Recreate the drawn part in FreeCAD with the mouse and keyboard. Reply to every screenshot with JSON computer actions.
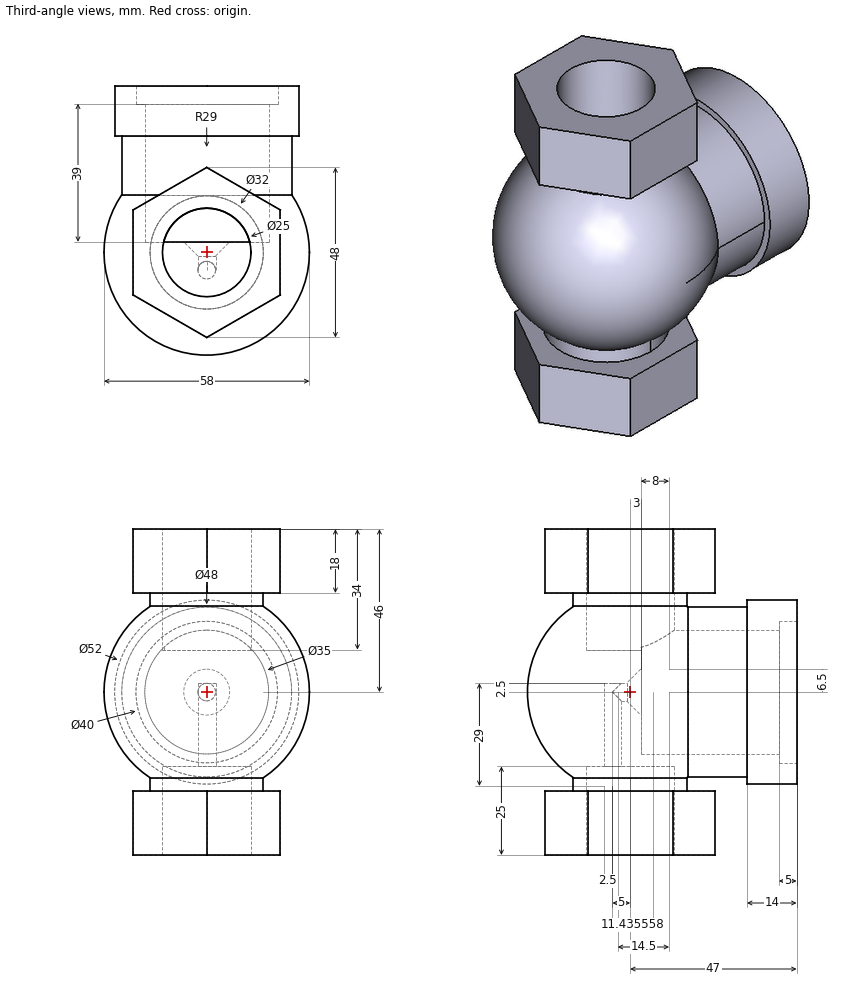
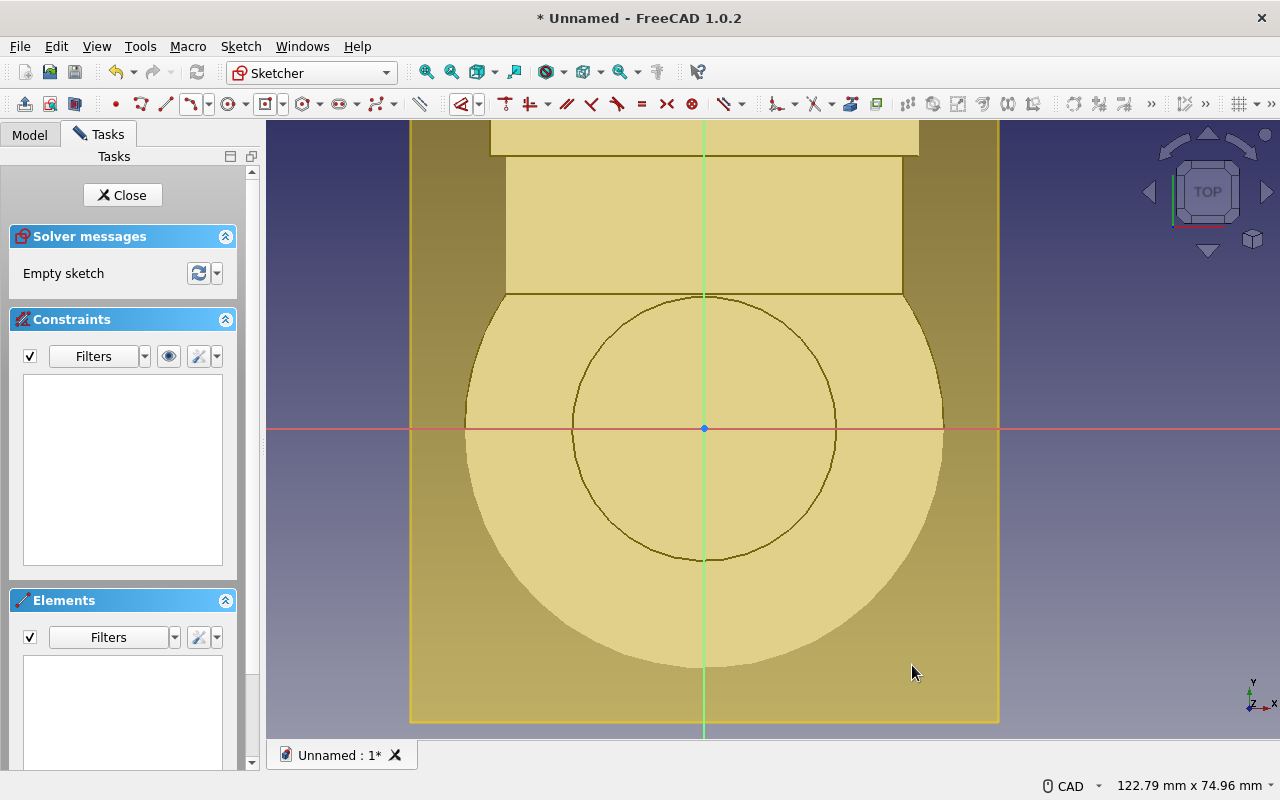
{"action": "left_click", "coordinate": [302, 104]}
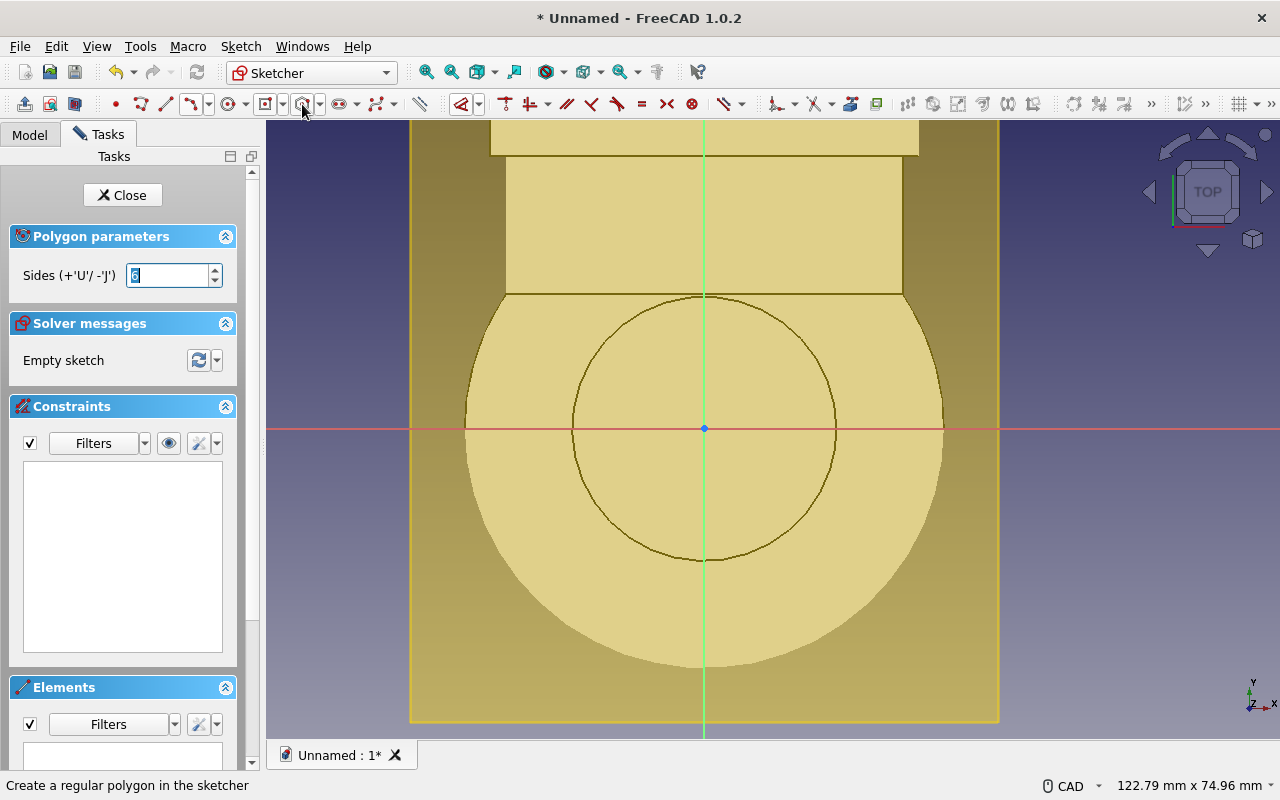
{"action": "left_click", "coordinate": [704, 429]}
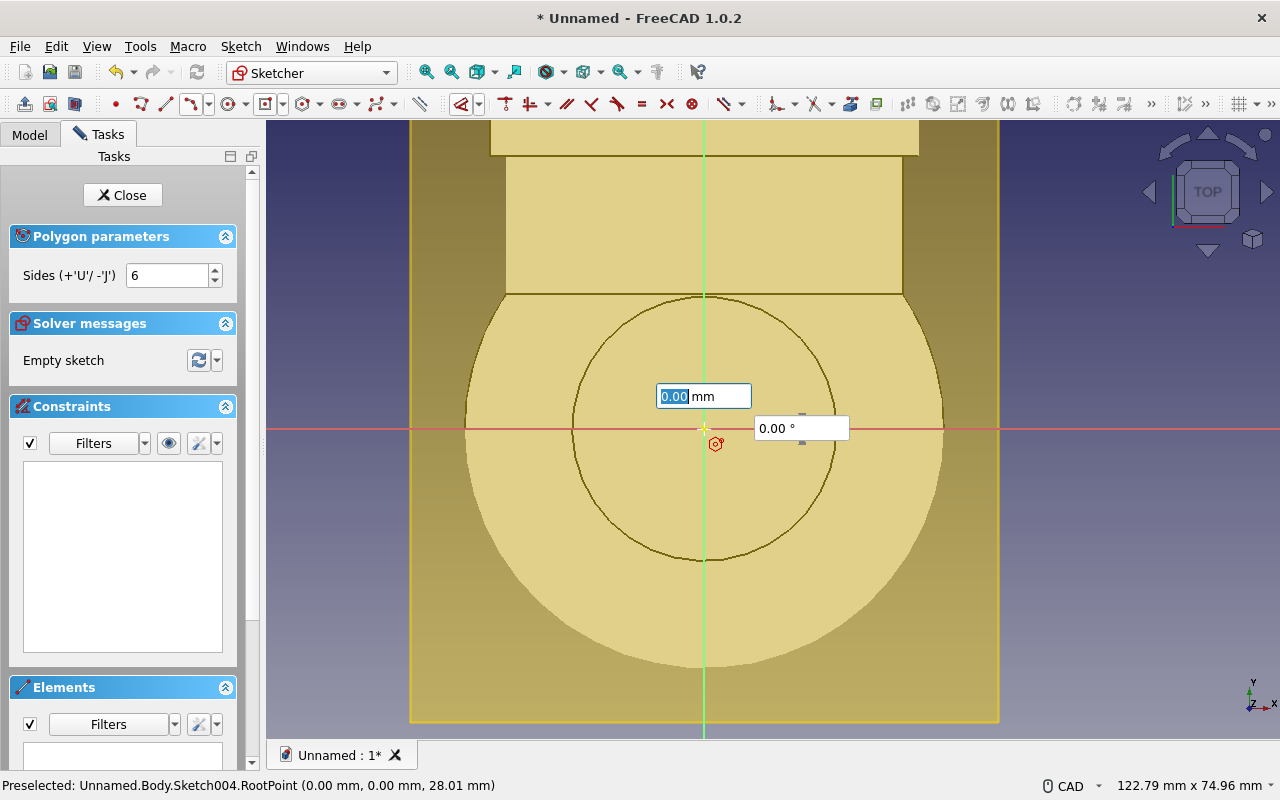
{"action": "left_click", "coordinate": [704, 231]}
{"action": "right_click", "coordinate": [704, 231]}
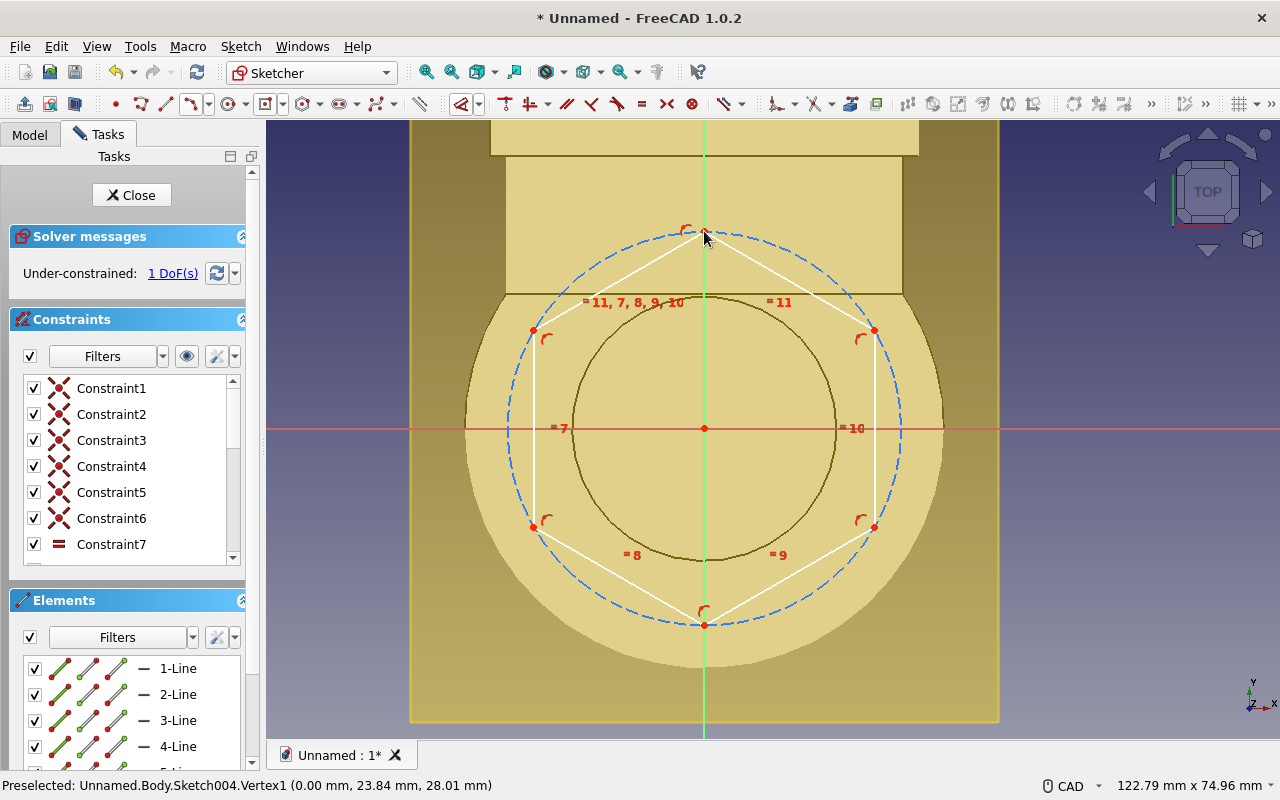
{"action": "left_click", "coordinate": [704, 626]}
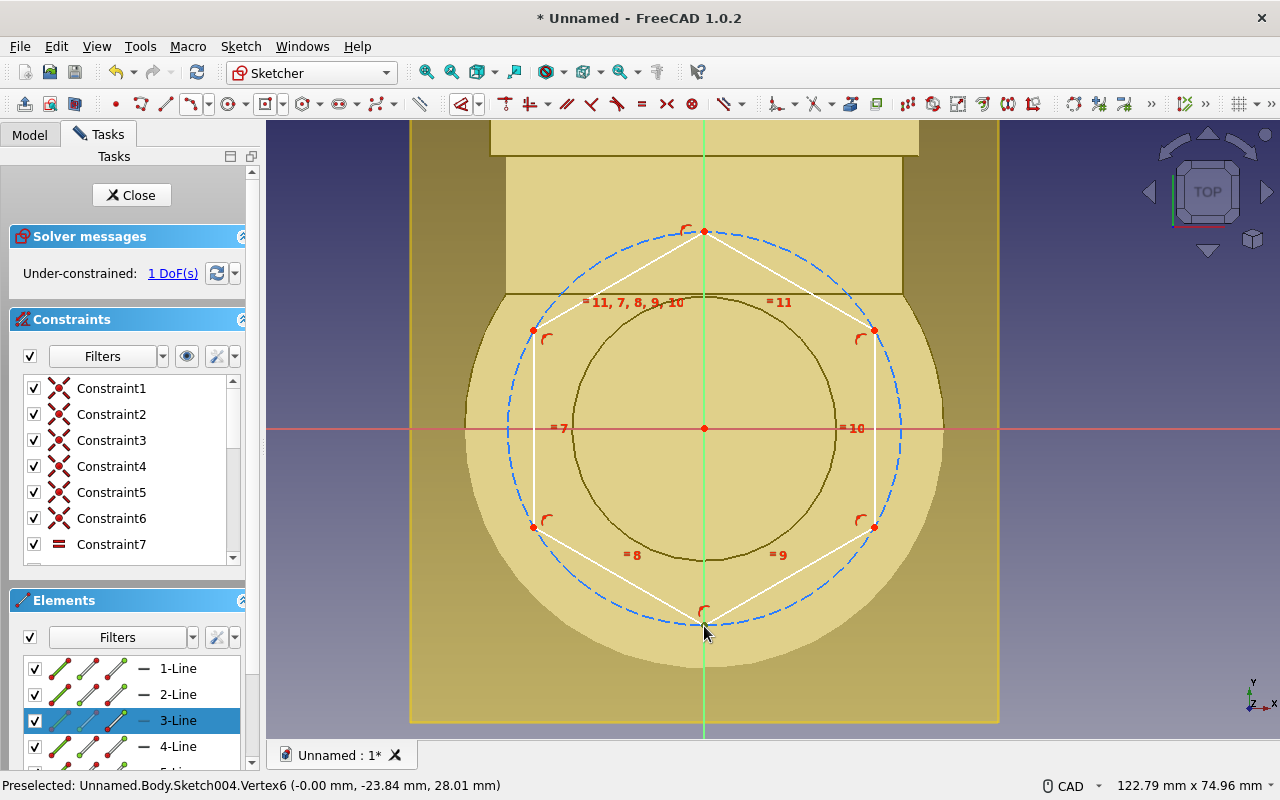
{"action": "left_click", "coordinate": [704, 232]}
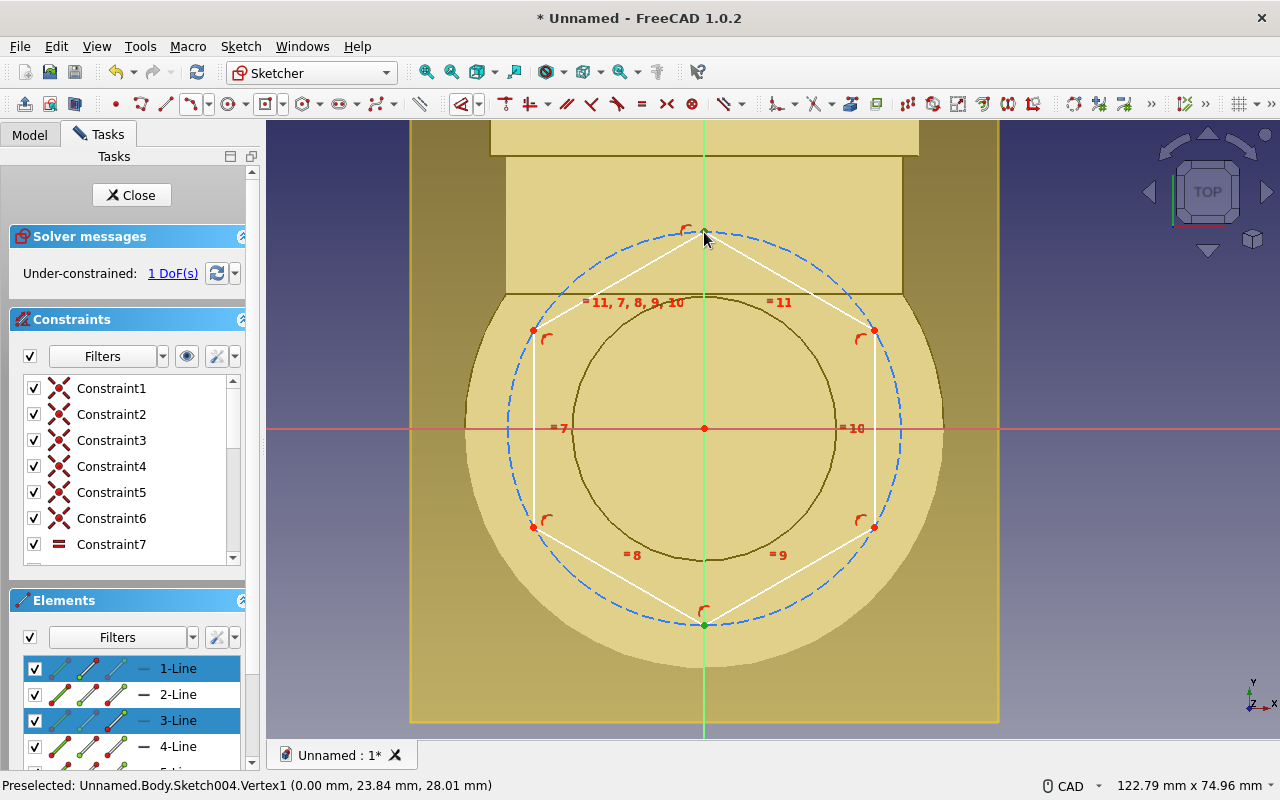
{"action": "key", "text": "i"}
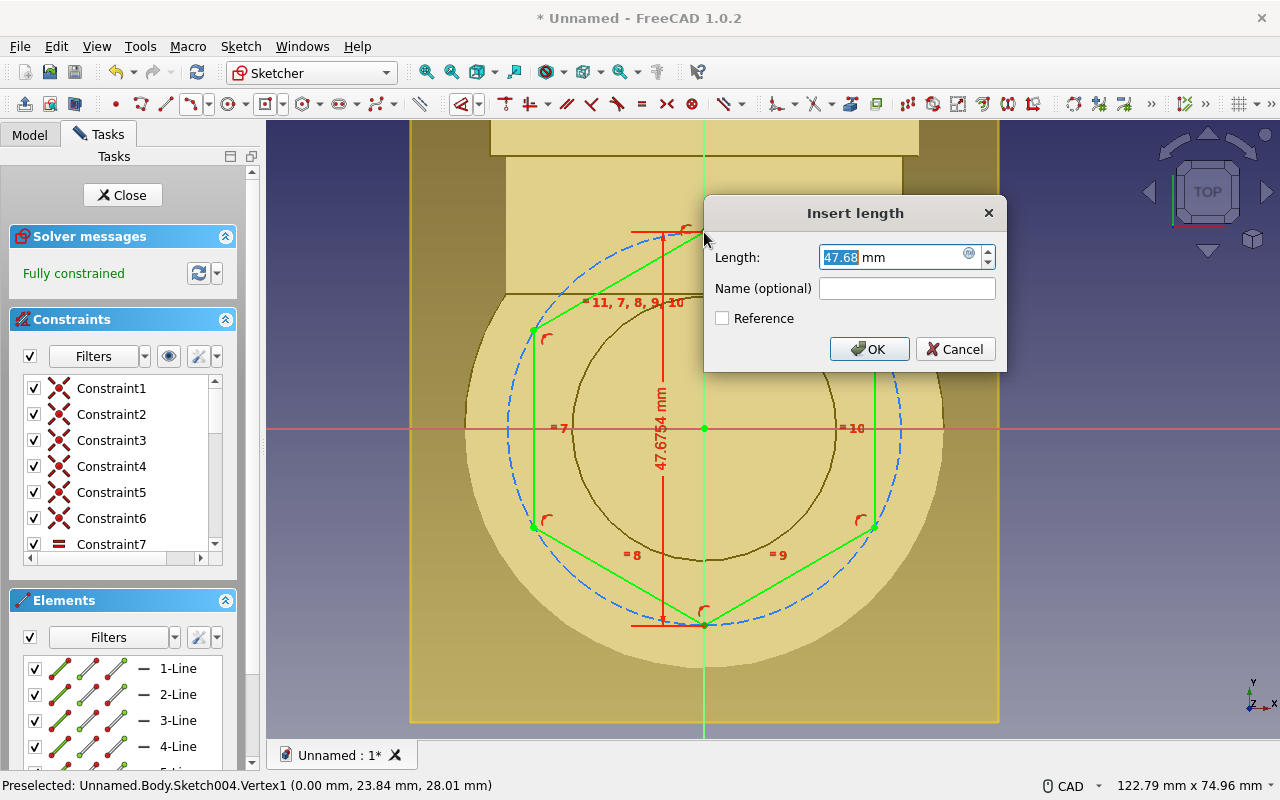
{"action": "type", "text": "48"}
{"action": "key", "text": "Return"}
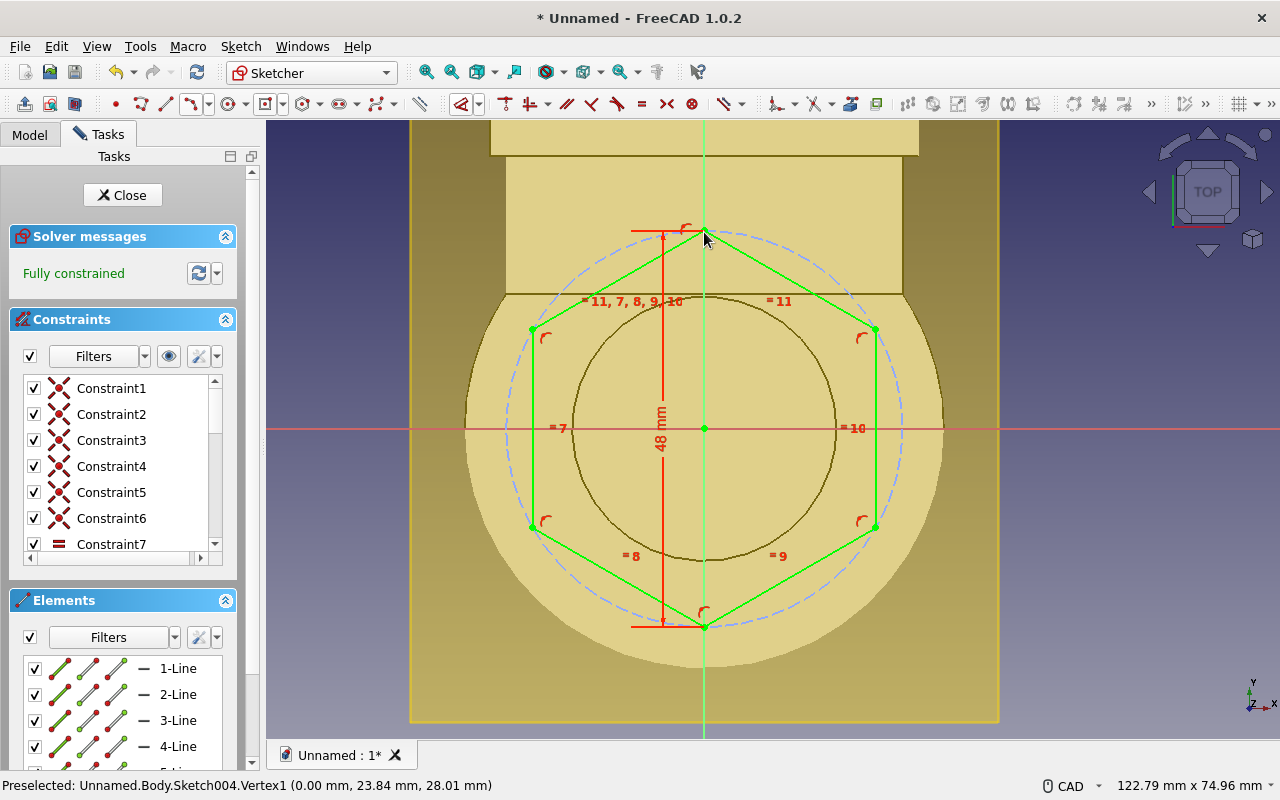
{"action": "left_click", "coordinate": [123, 195]}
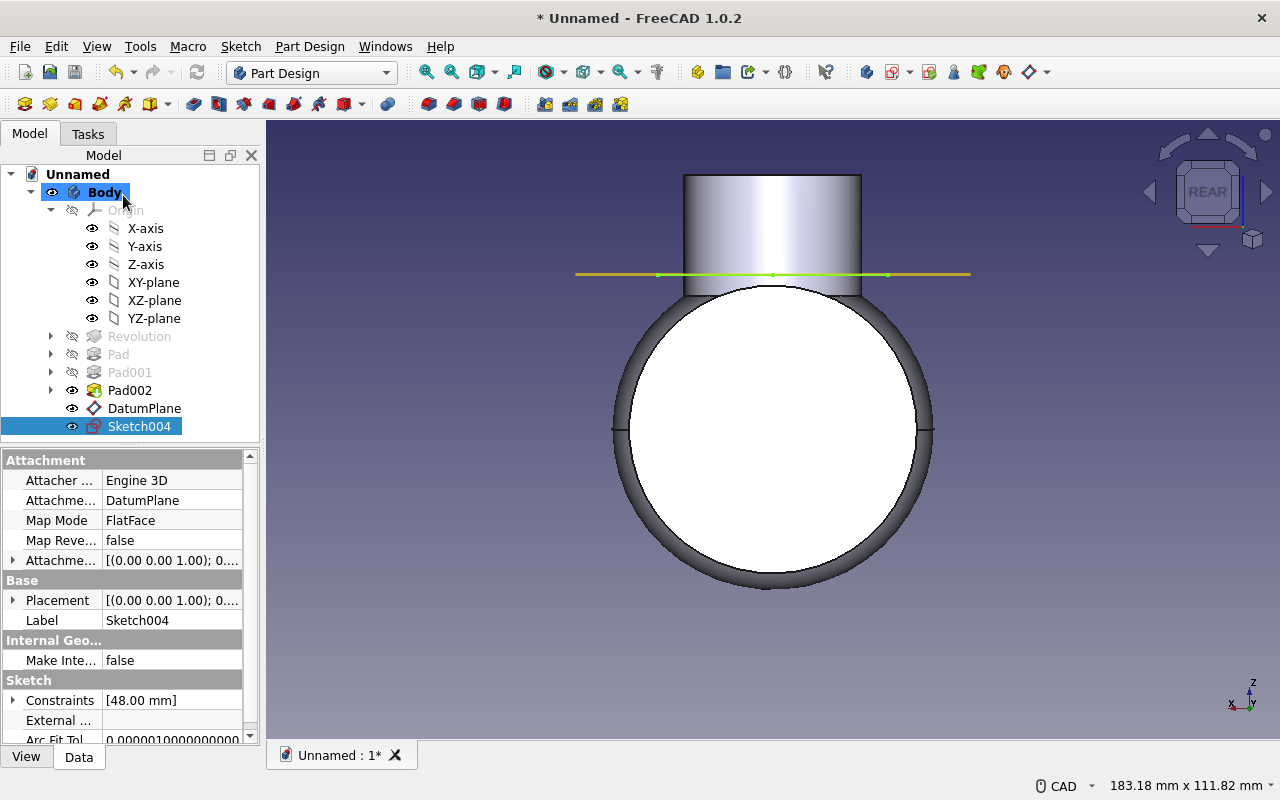
{"action": "left_click", "coordinate": [25, 104]}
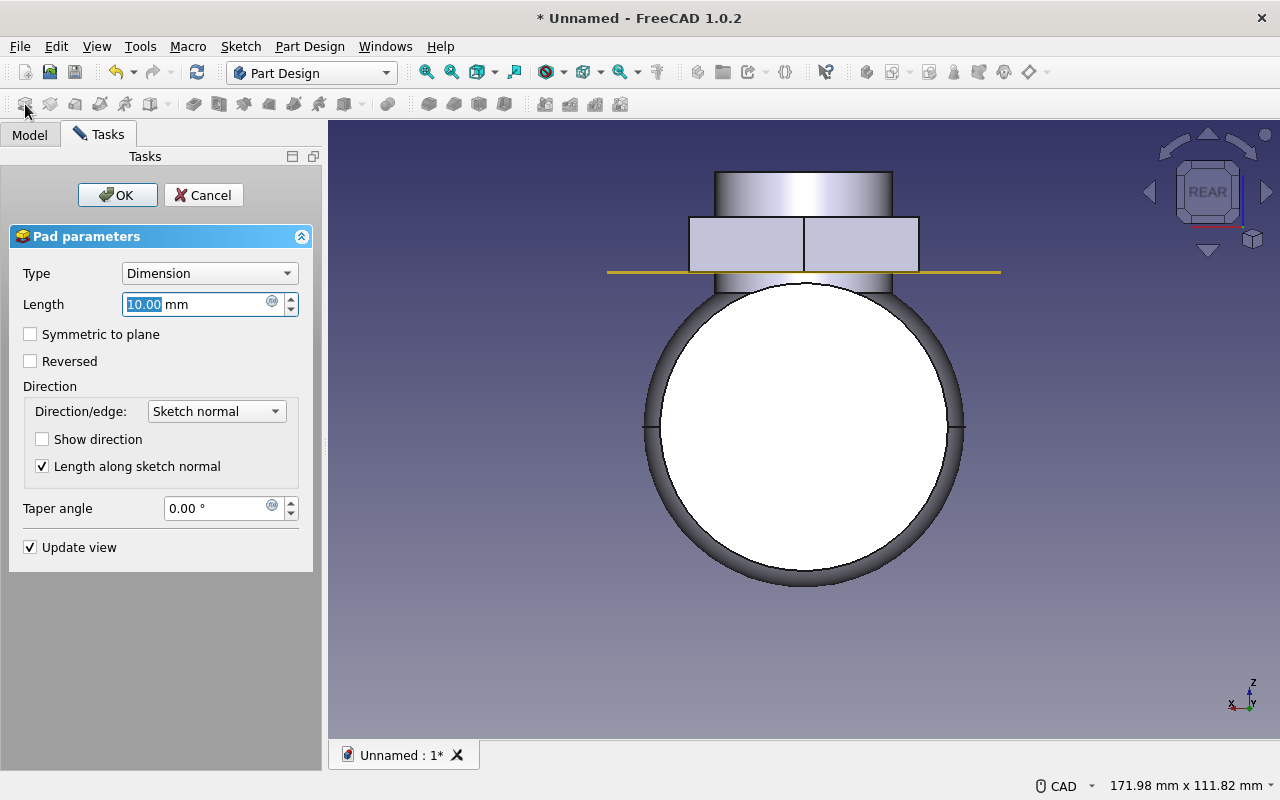
{"action": "type", "text": "18"}
{"action": "key", "text": "Tab"}